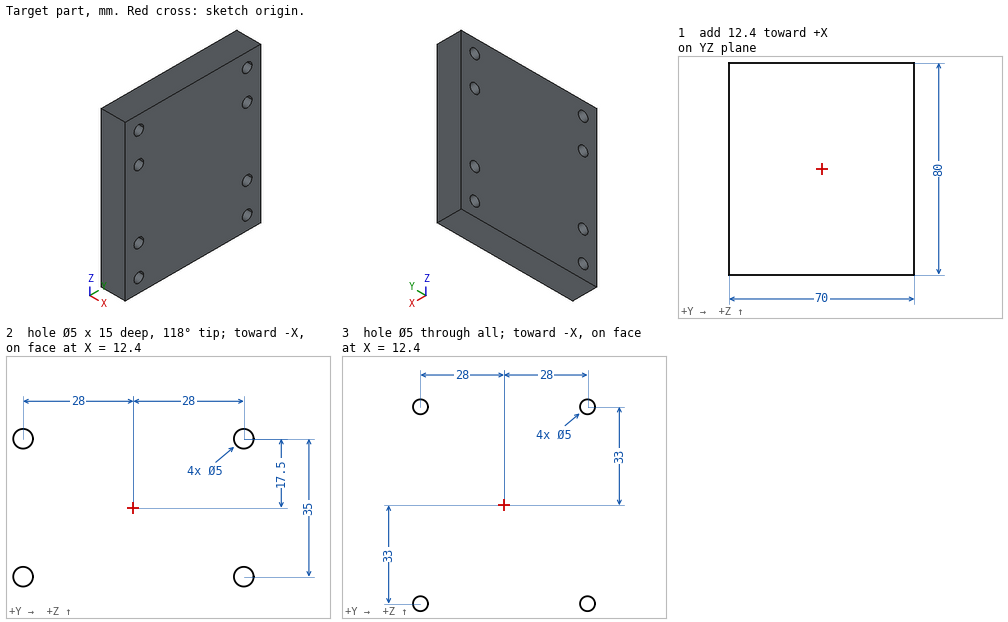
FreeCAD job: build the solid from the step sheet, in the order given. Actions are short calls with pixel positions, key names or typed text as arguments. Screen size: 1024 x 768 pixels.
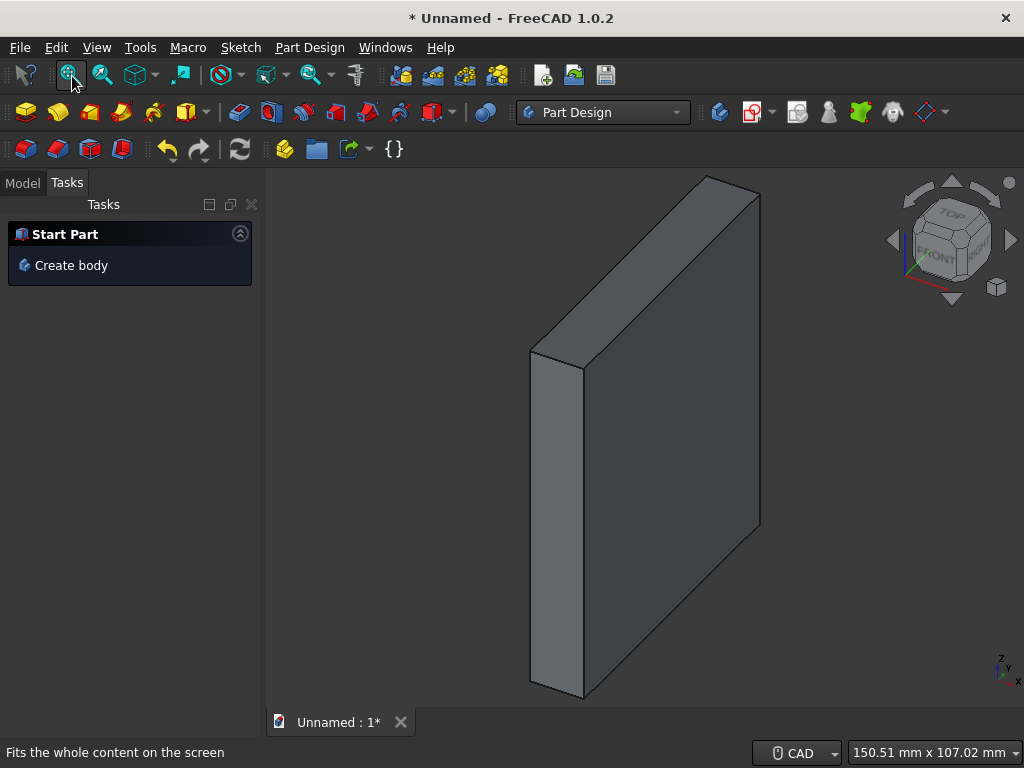
click(672, 445)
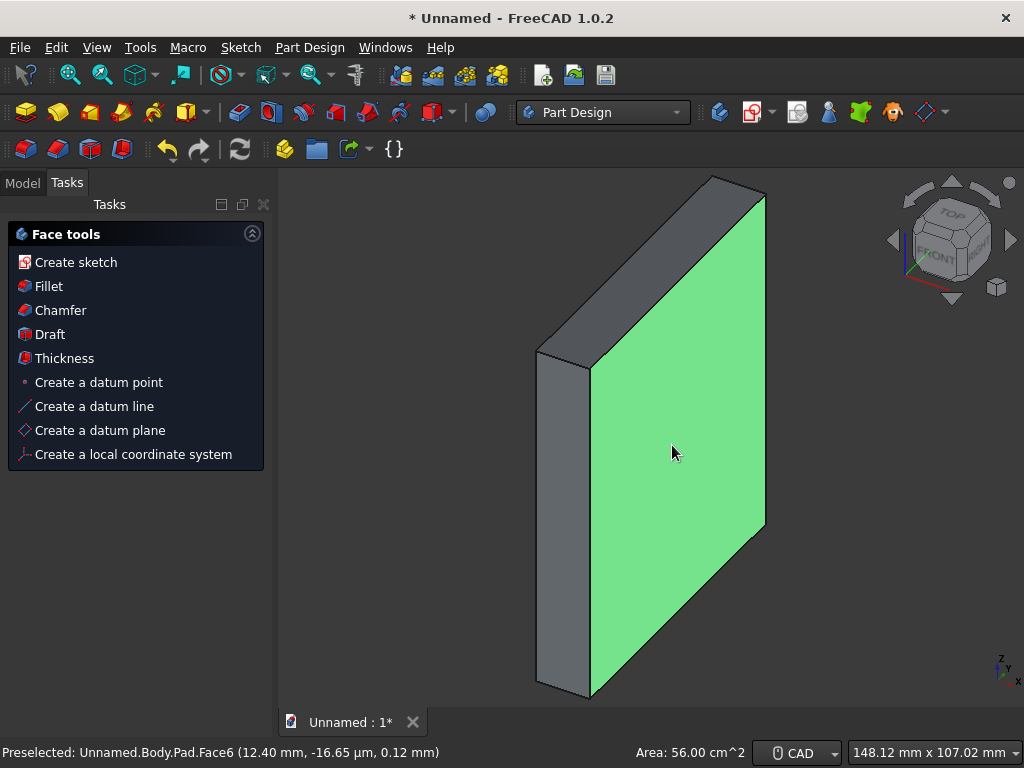
click(752, 112)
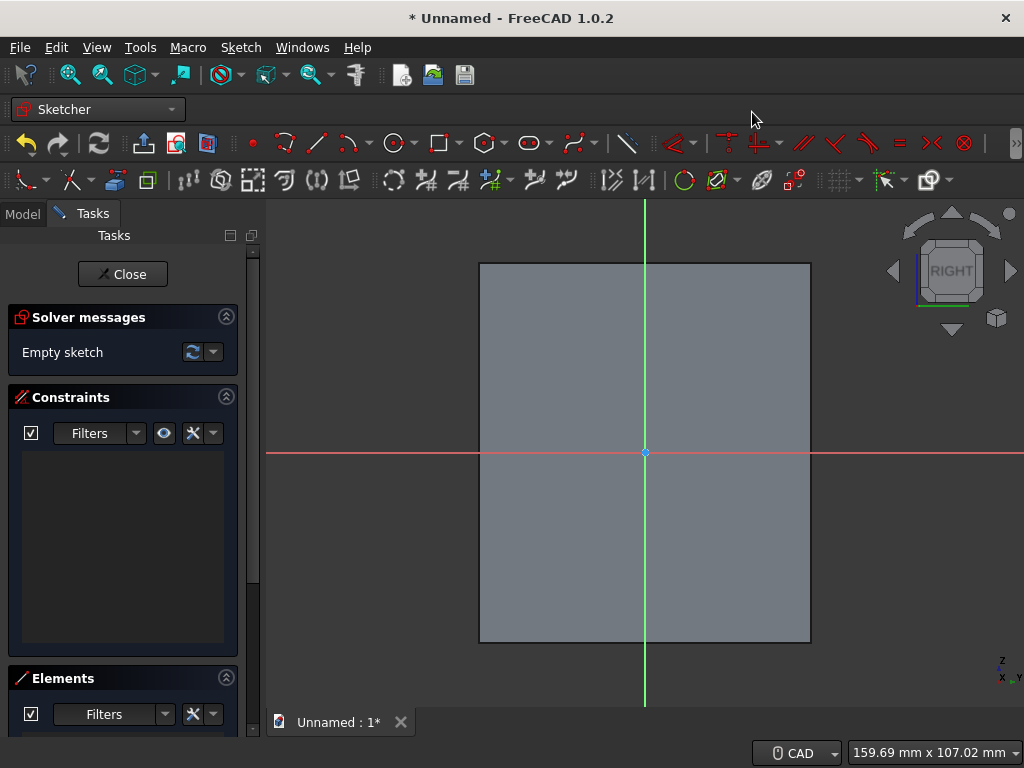
scroll(784, 453, up, 2)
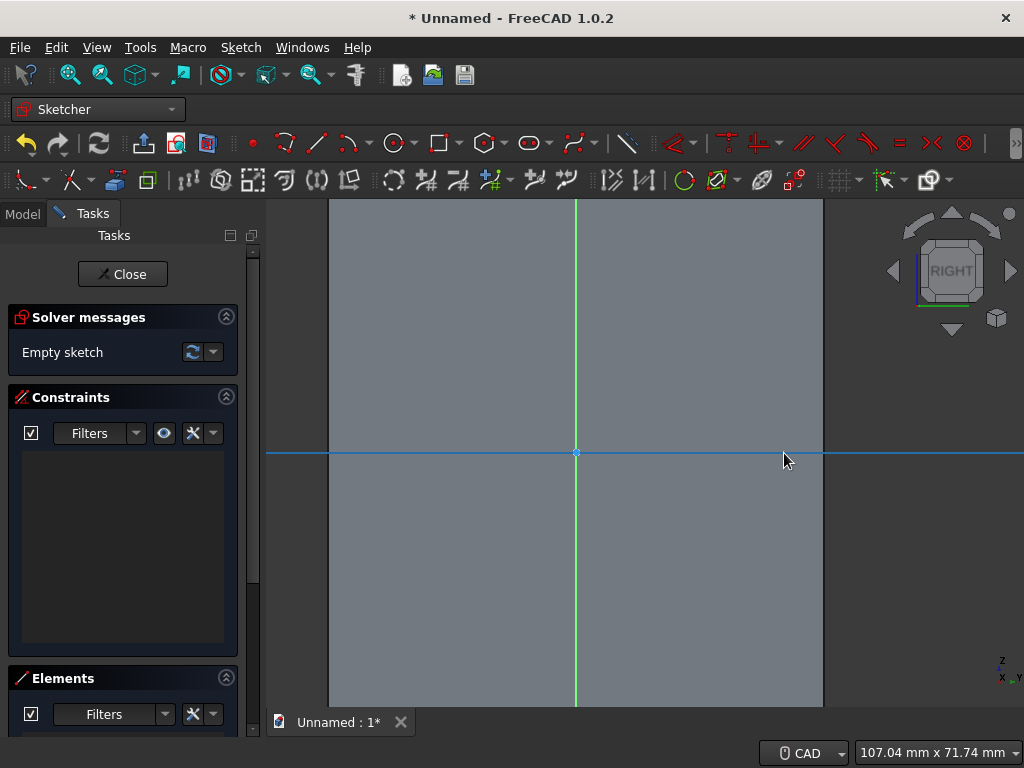
click(394, 144)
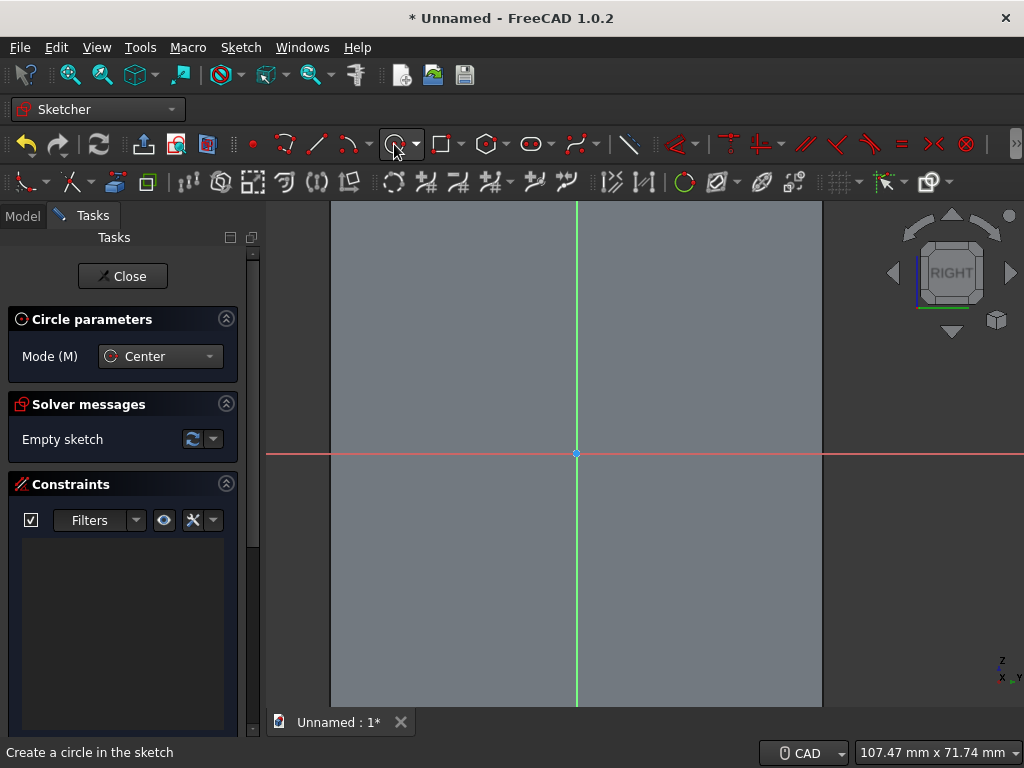
scroll(774, 330, up, 2)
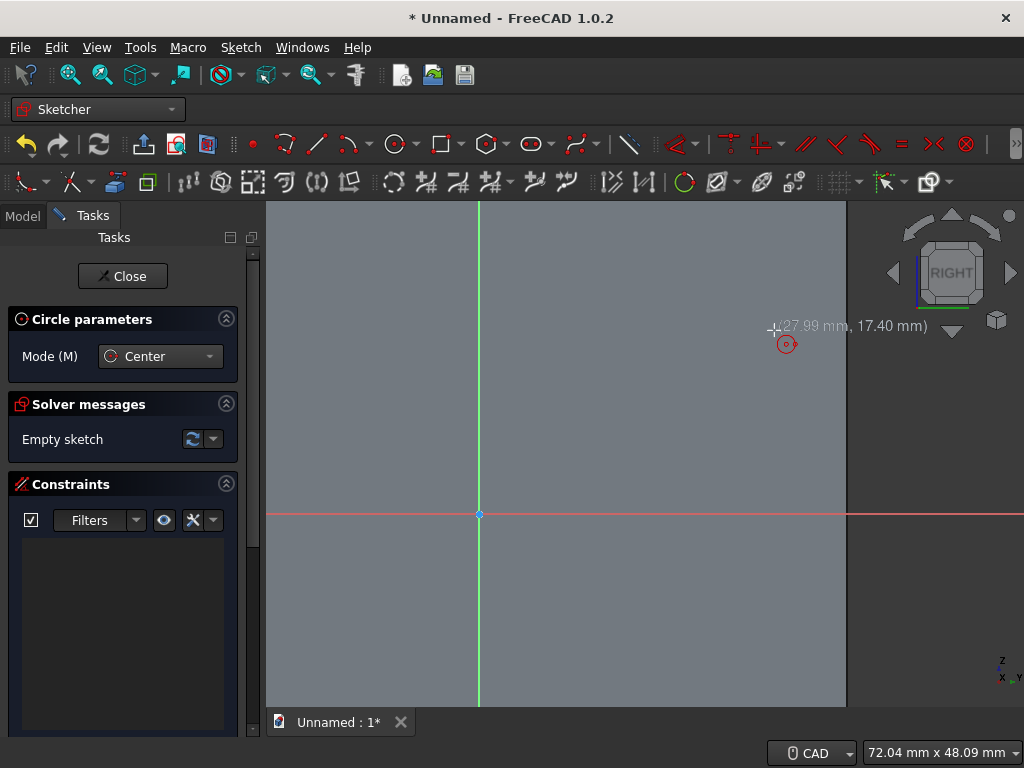
click(774, 330)
move(792, 312)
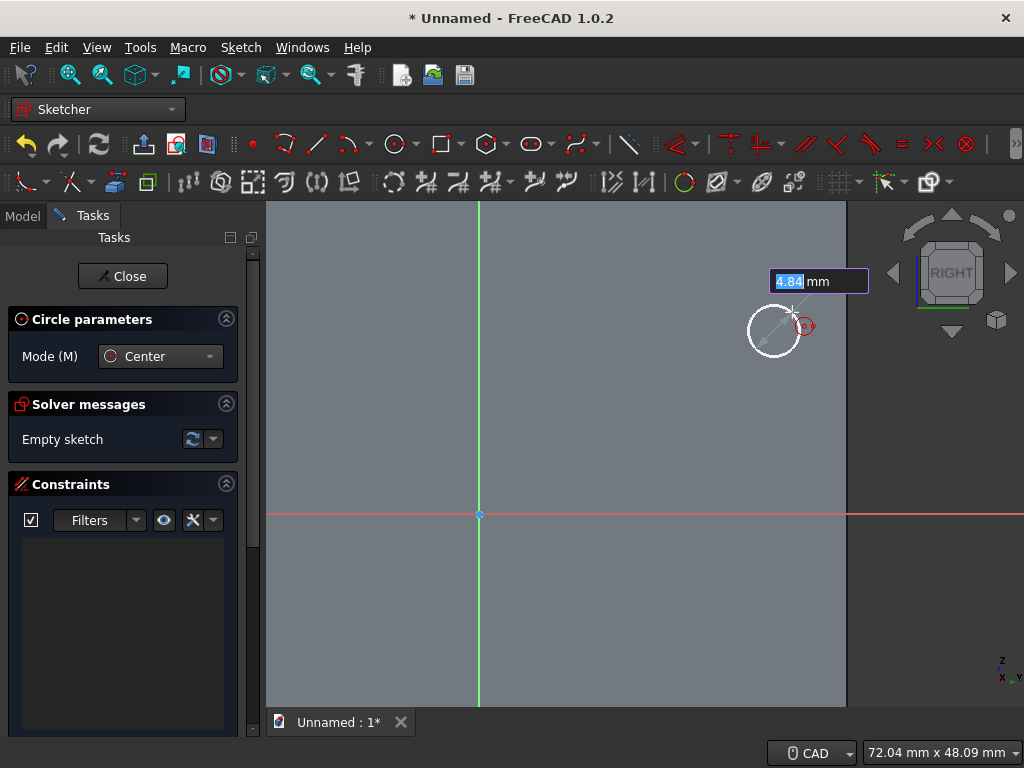
text(5)
key(Return)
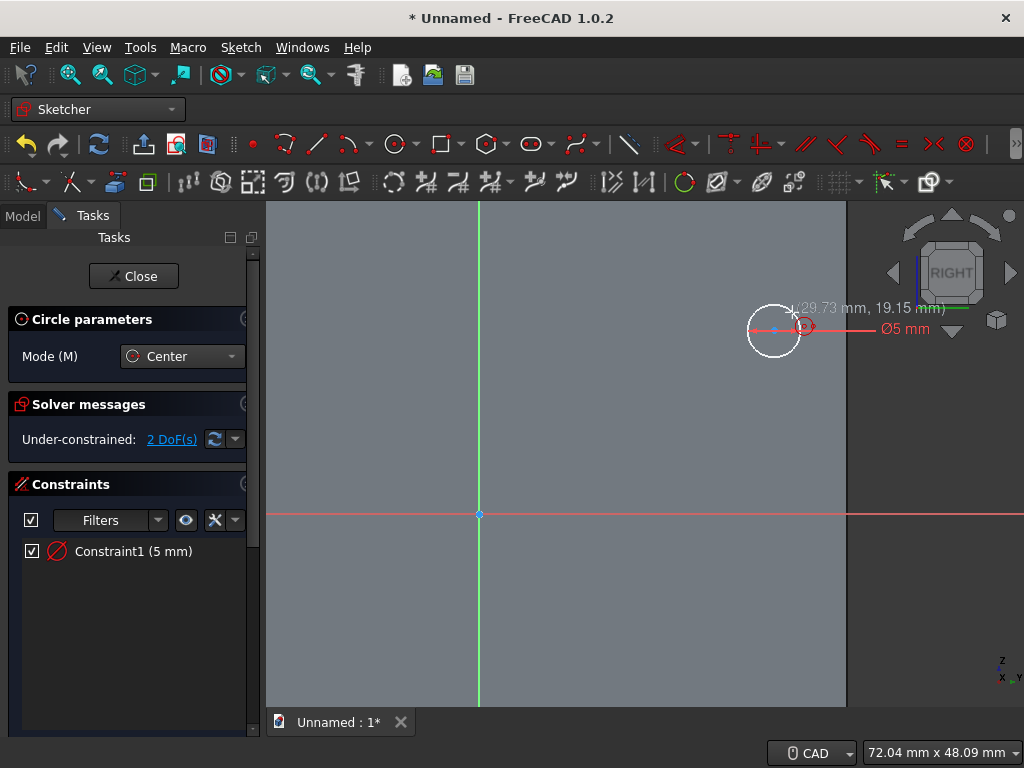
scroll(774, 331, down, 2)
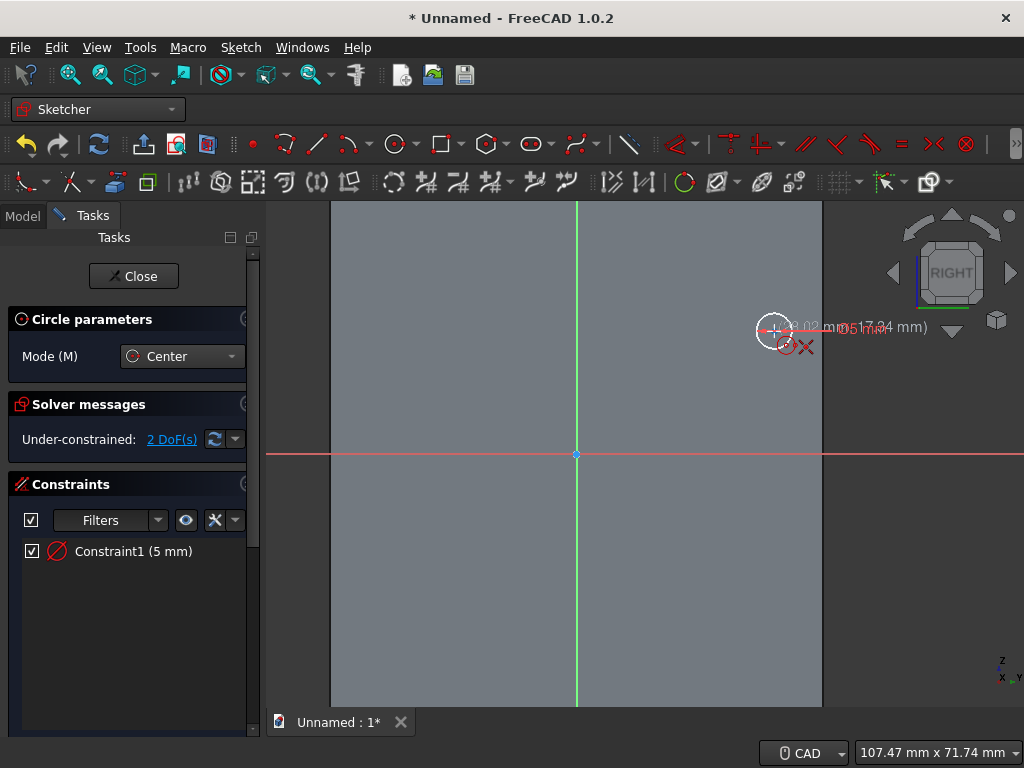
scroll(774, 578, up, 2)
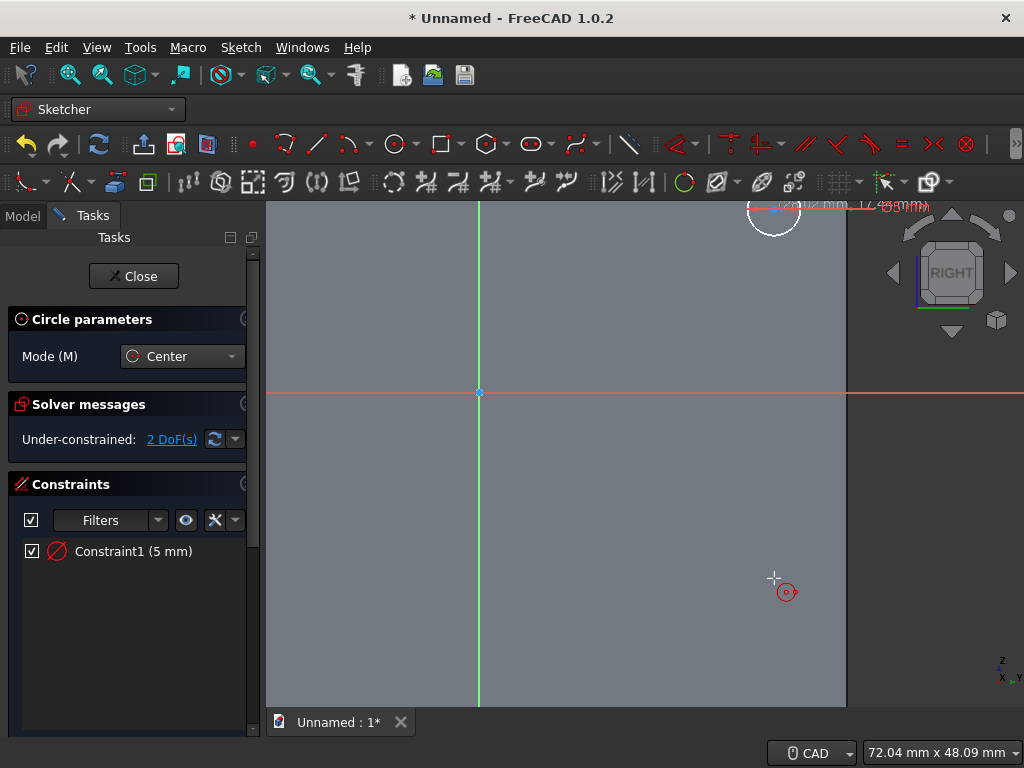
click(774, 577)
move(792, 558)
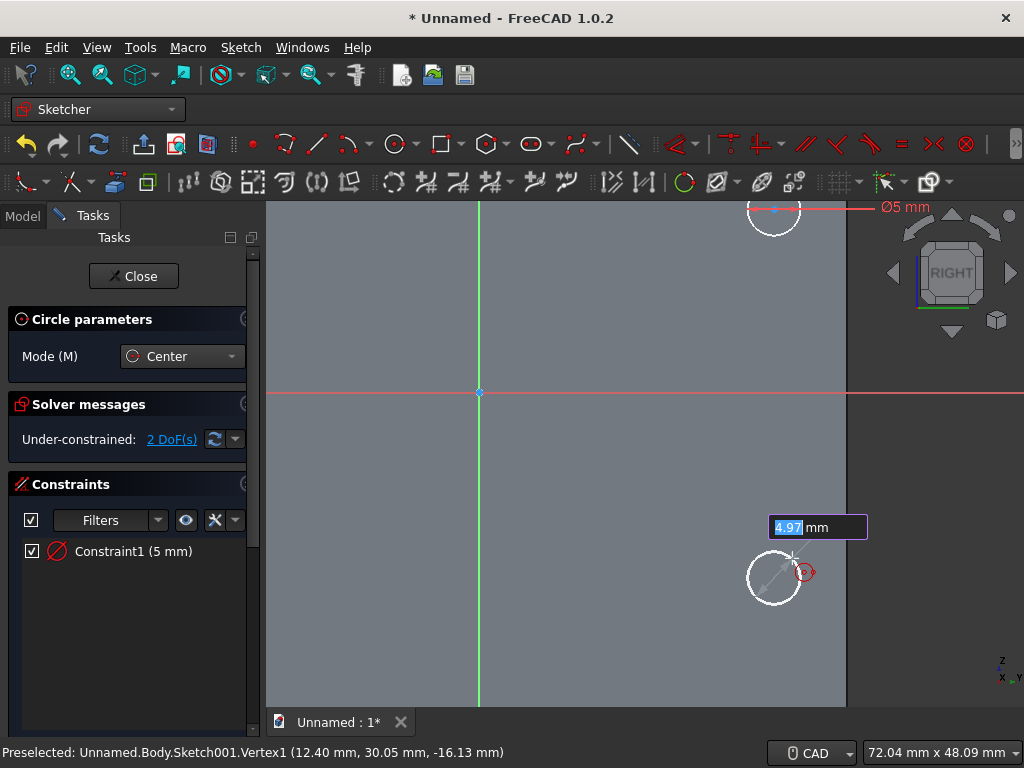
text(5)
key(Return)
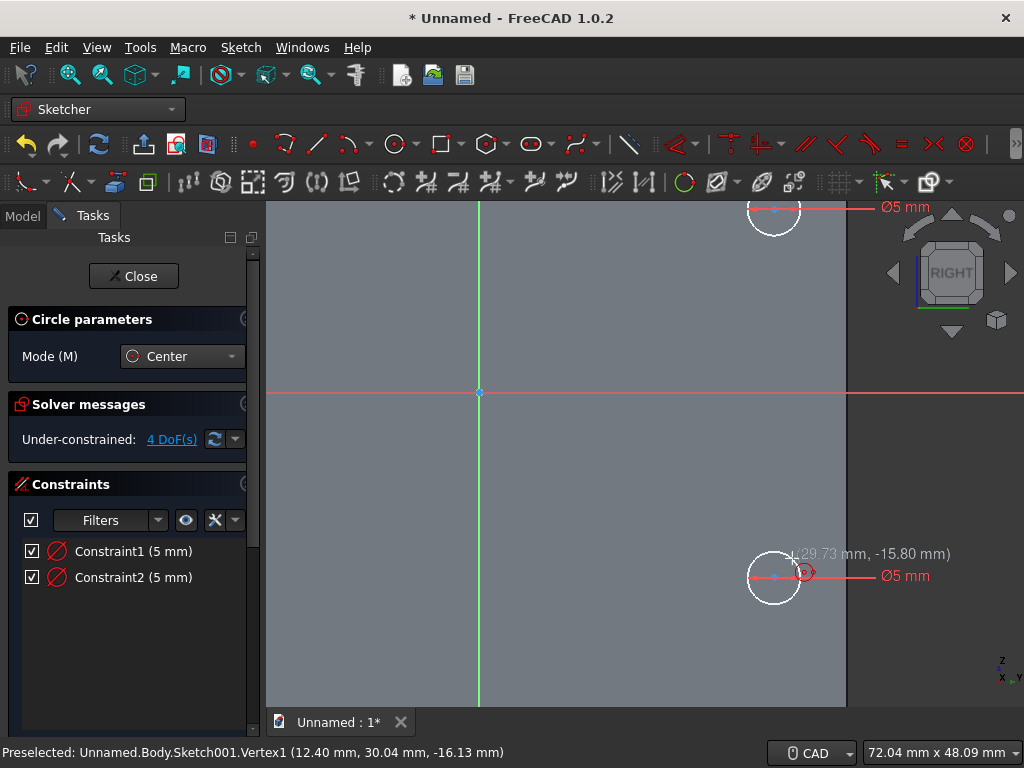
scroll(774, 578, down, 2)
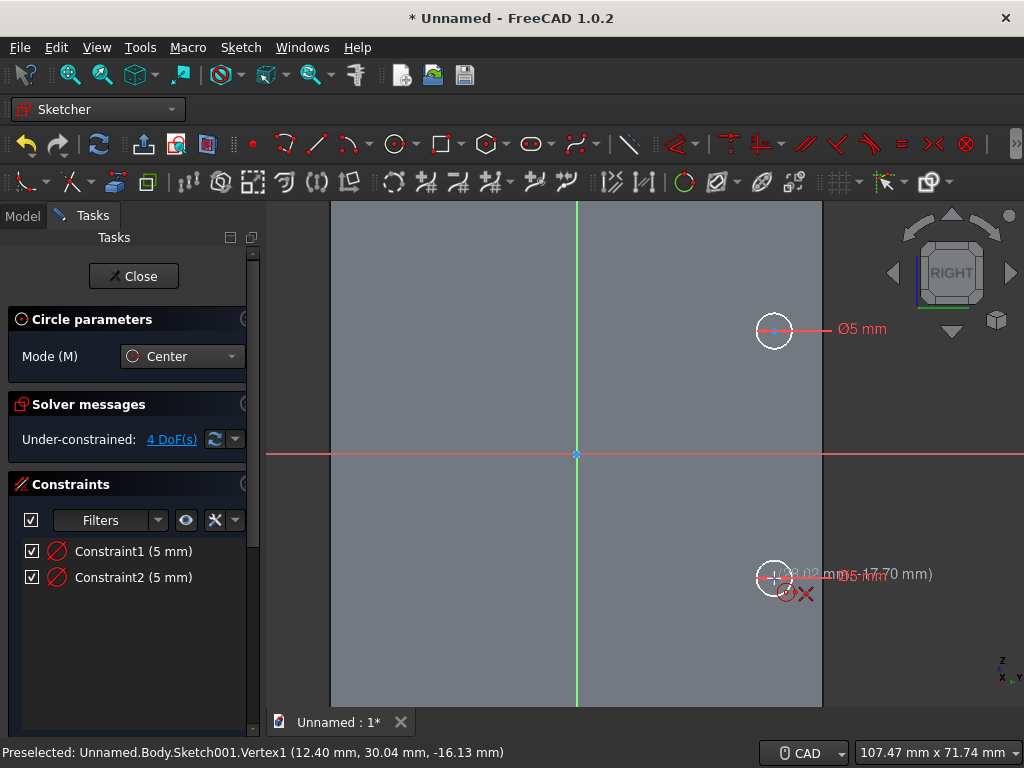
scroll(379, 331, up, 2)